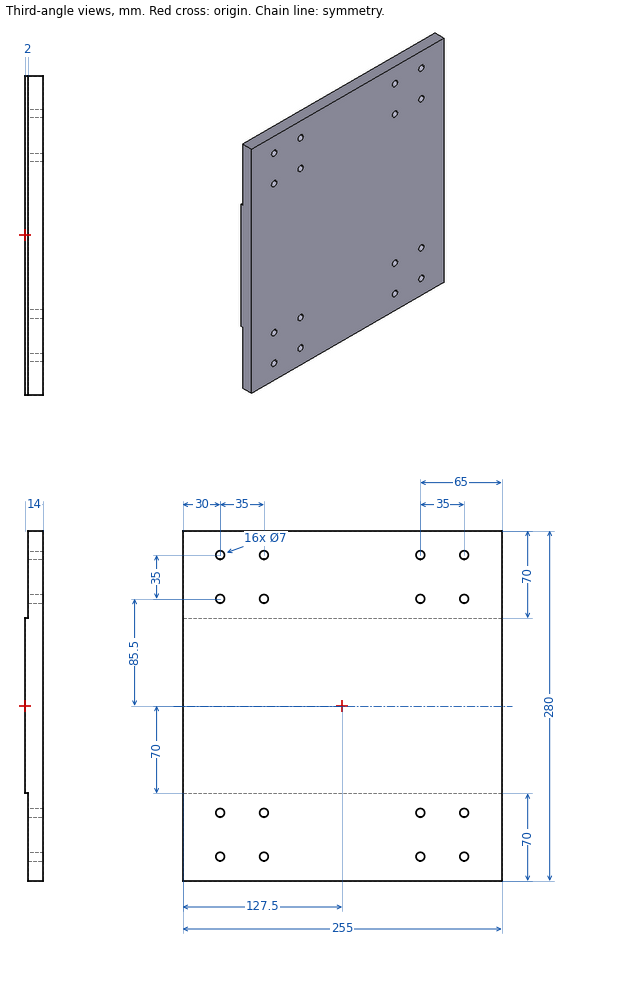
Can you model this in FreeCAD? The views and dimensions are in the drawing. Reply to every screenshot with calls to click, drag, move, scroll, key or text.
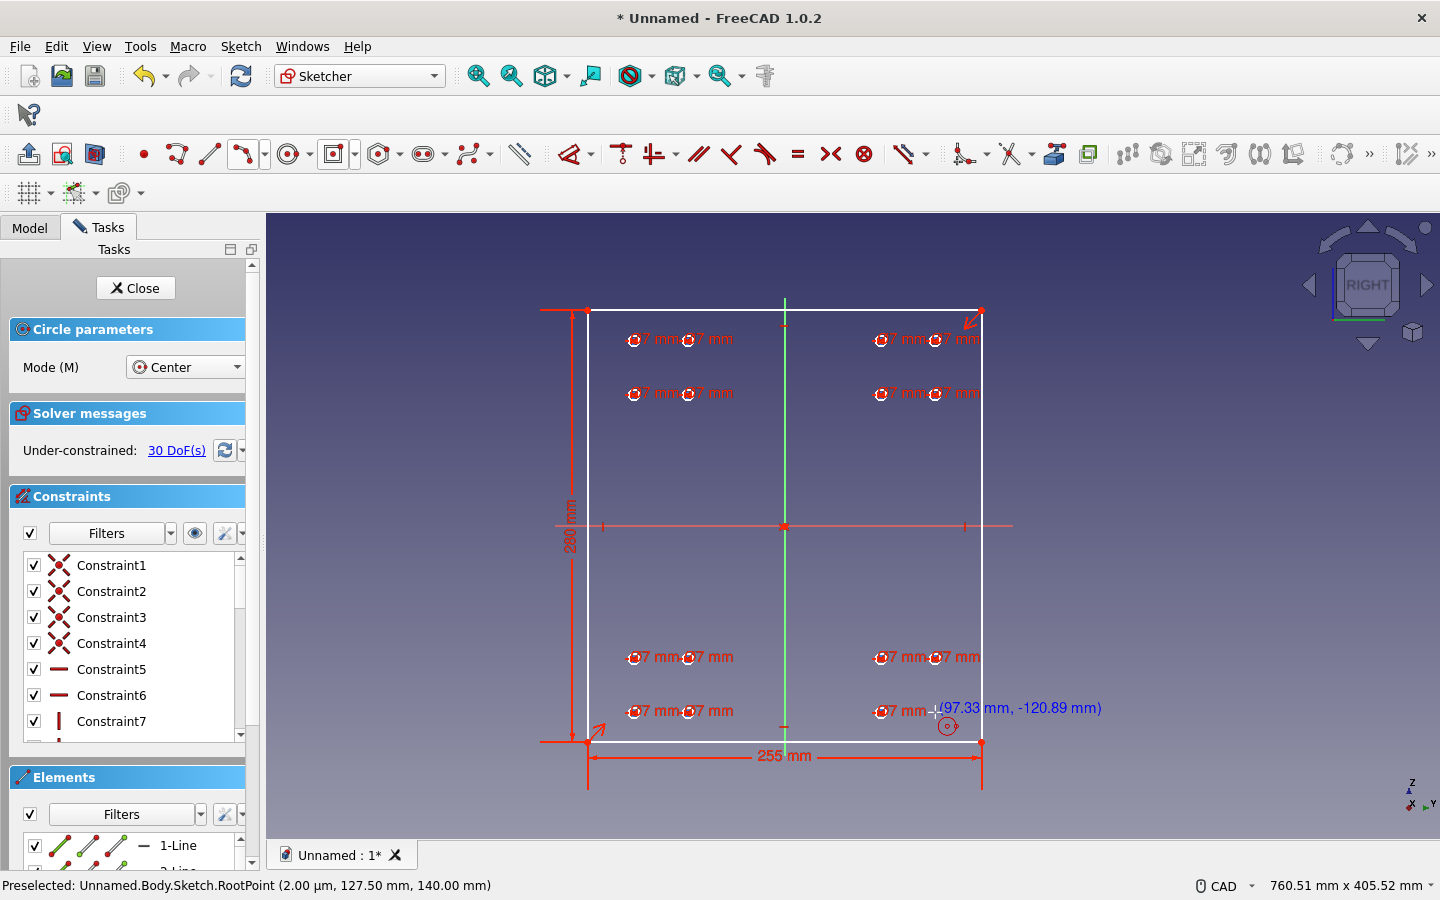
click(935, 712)
move(939, 709)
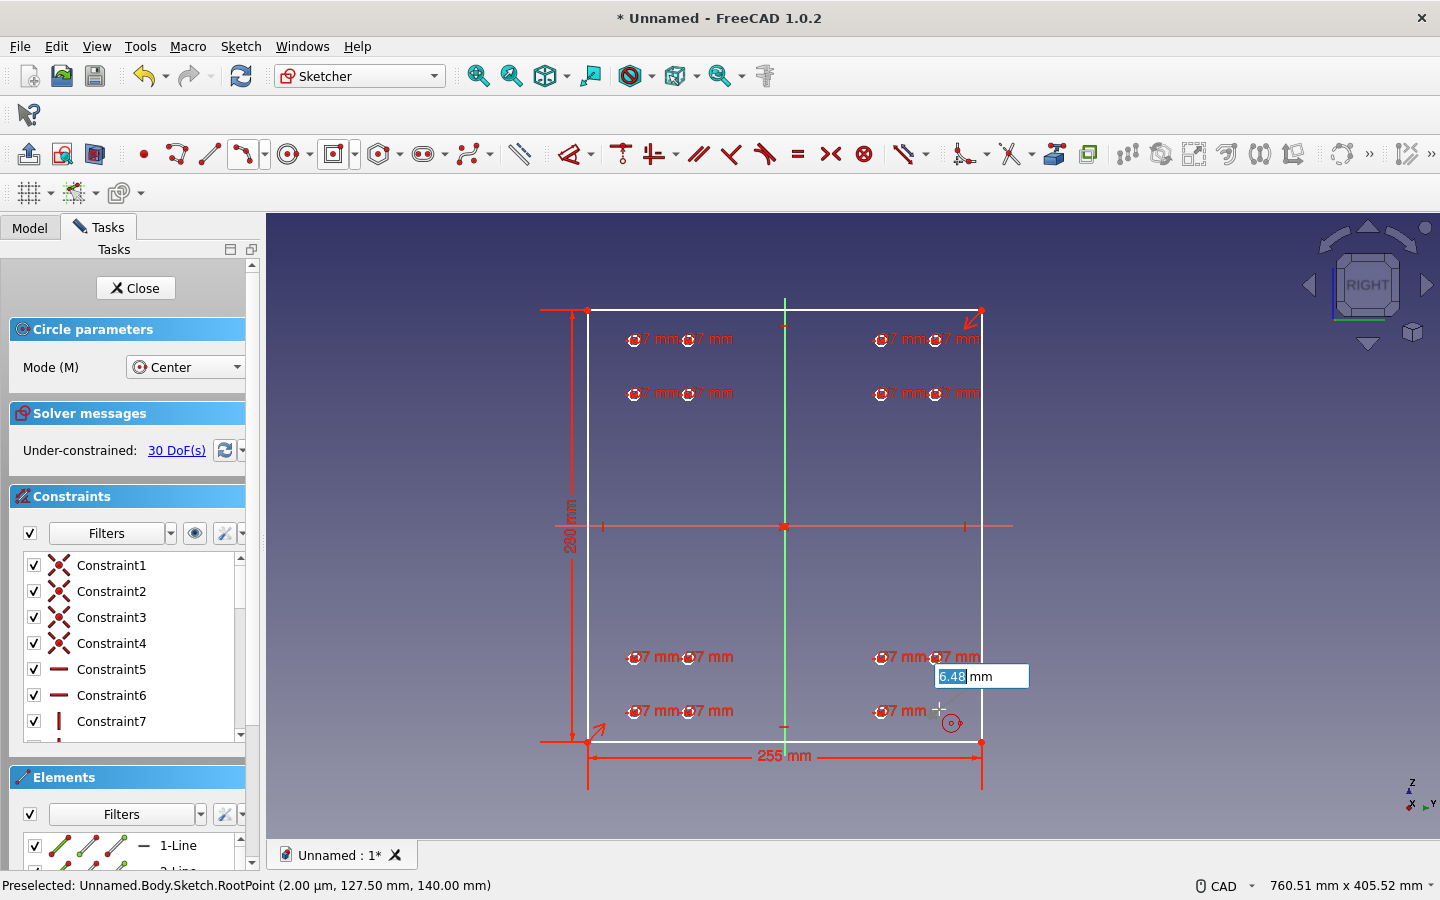
text(7)
key(Return)
key(Escape)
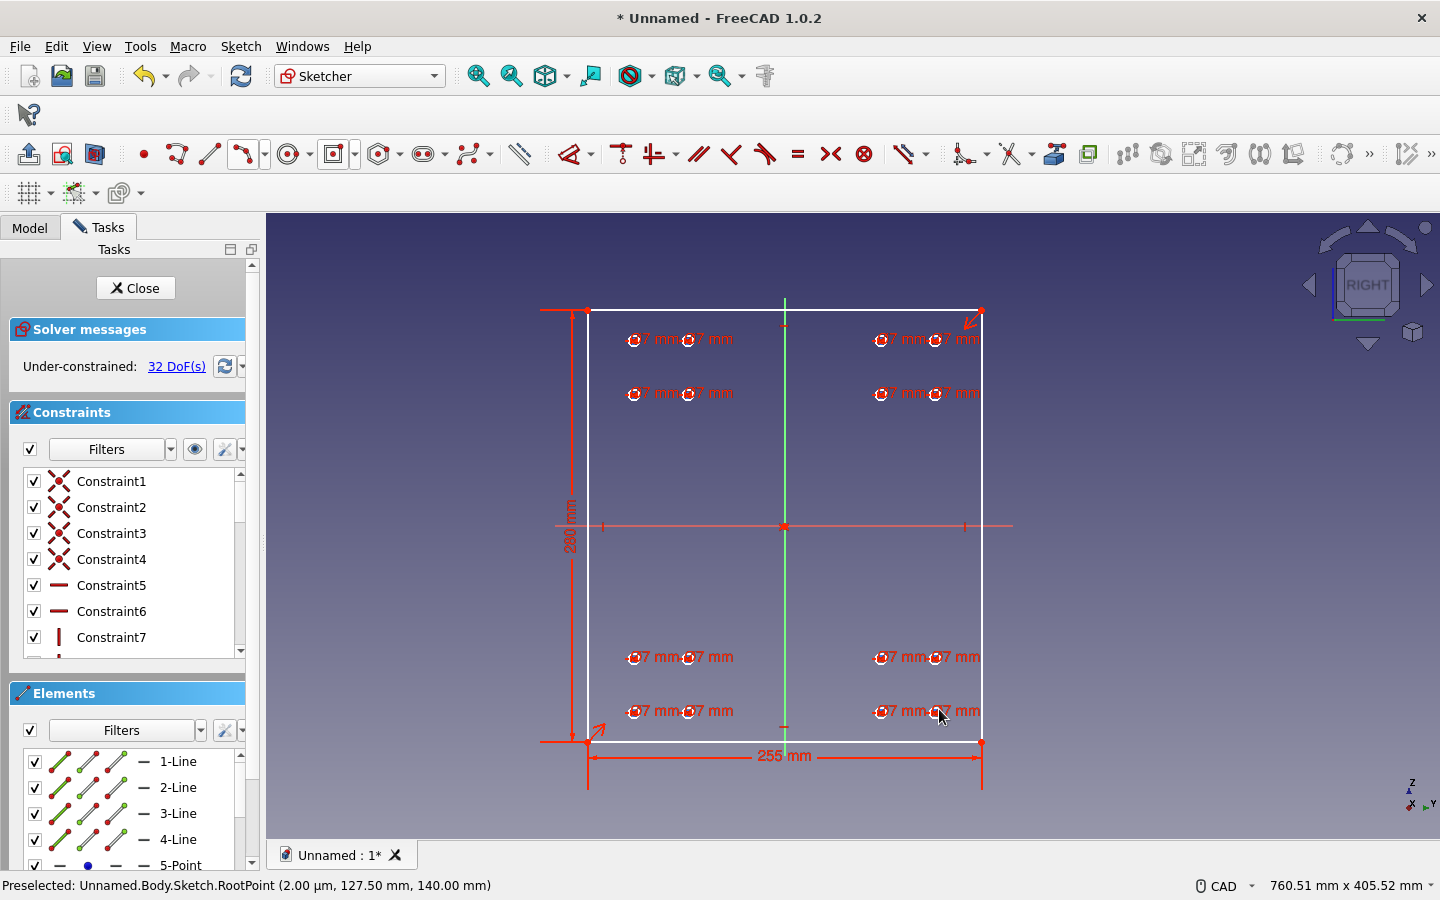
click(634, 341)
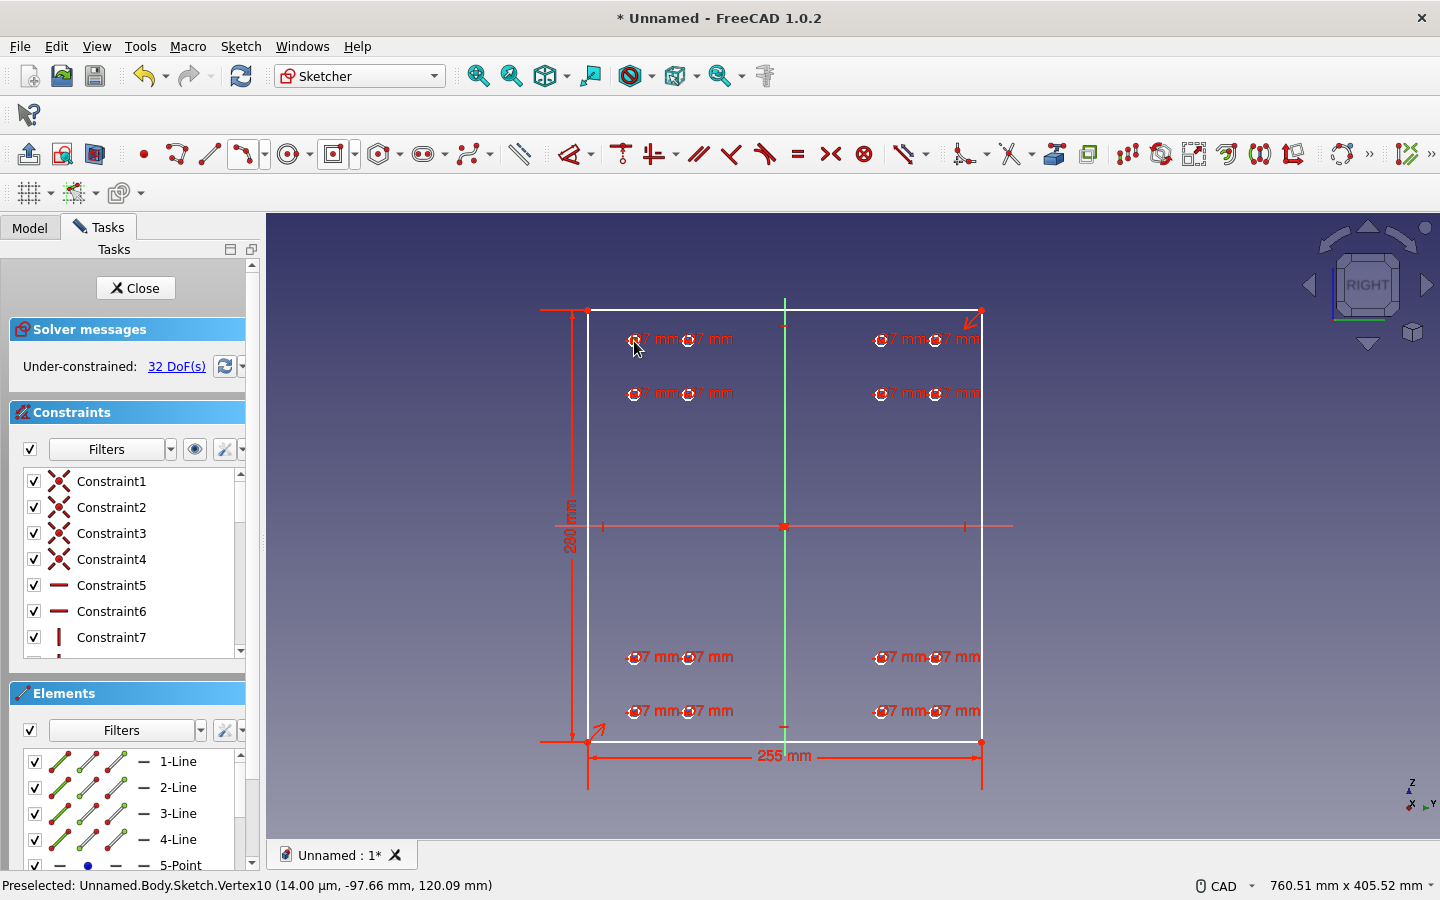
click(634, 395)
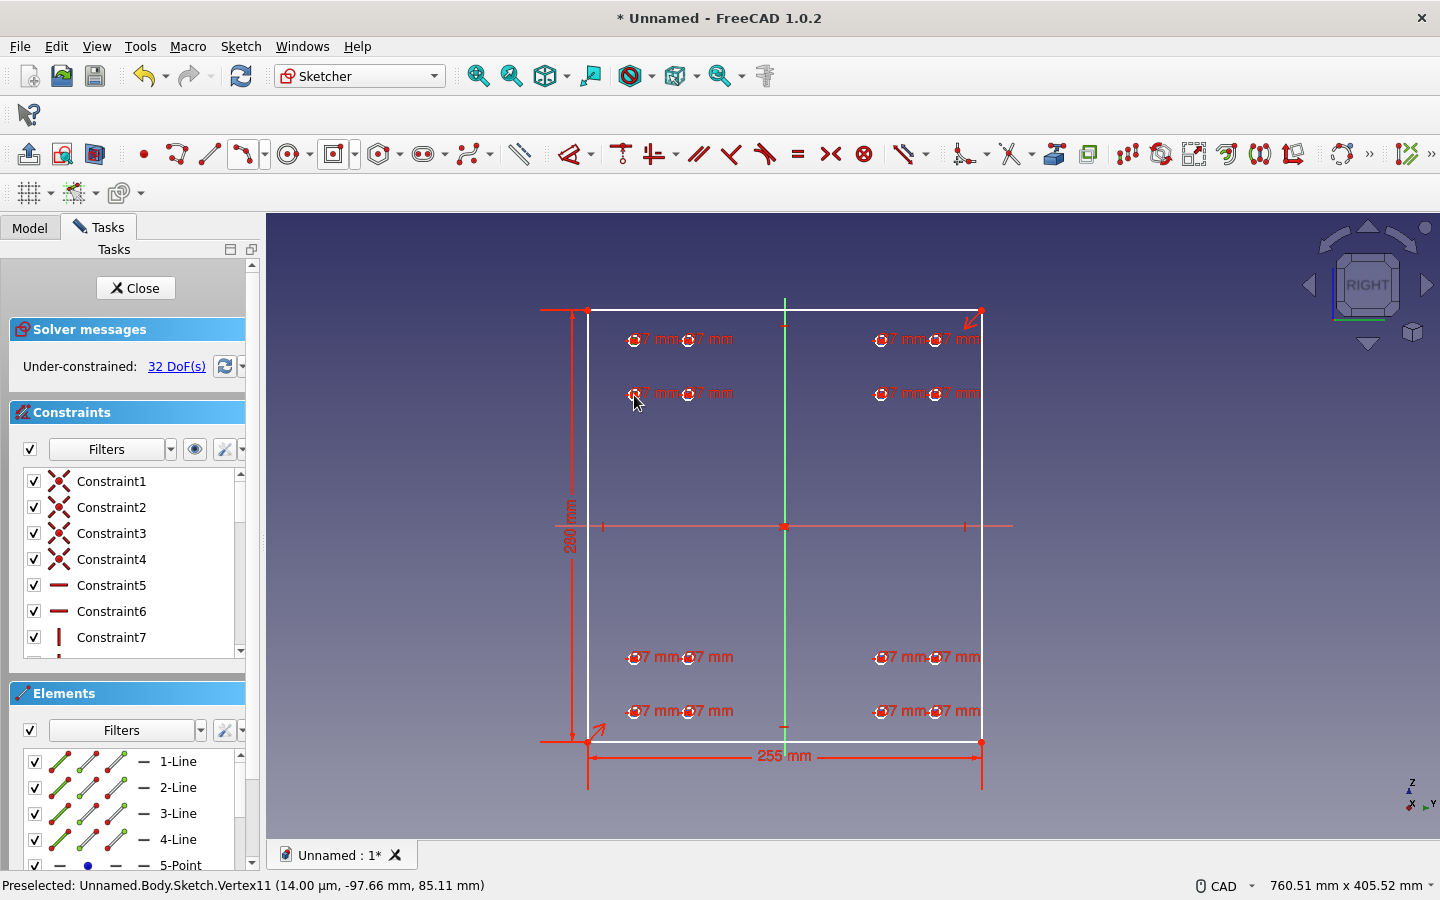
click(676, 154)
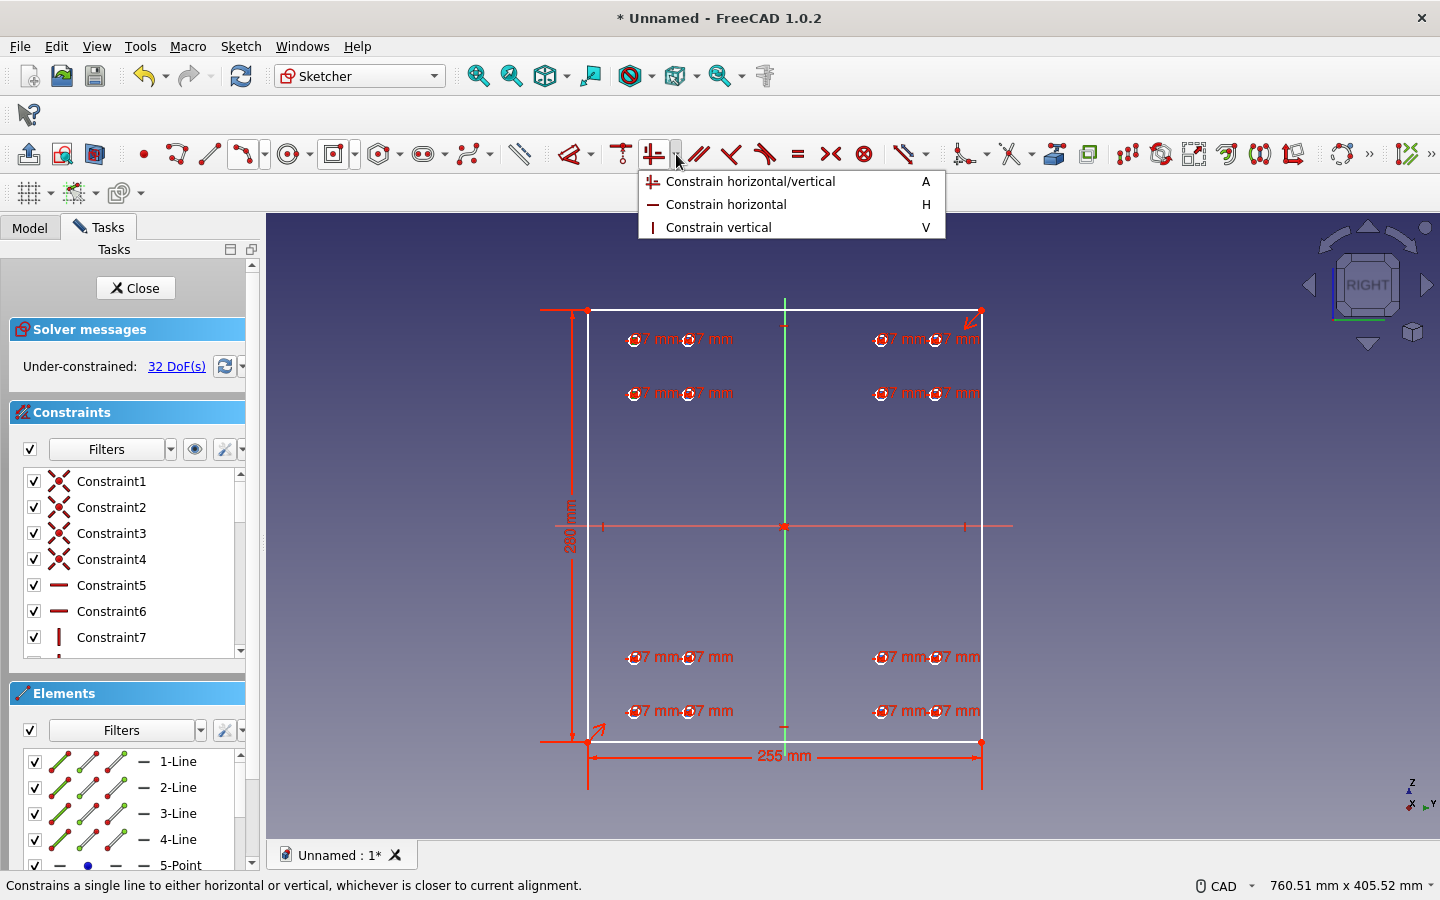
click(792, 228)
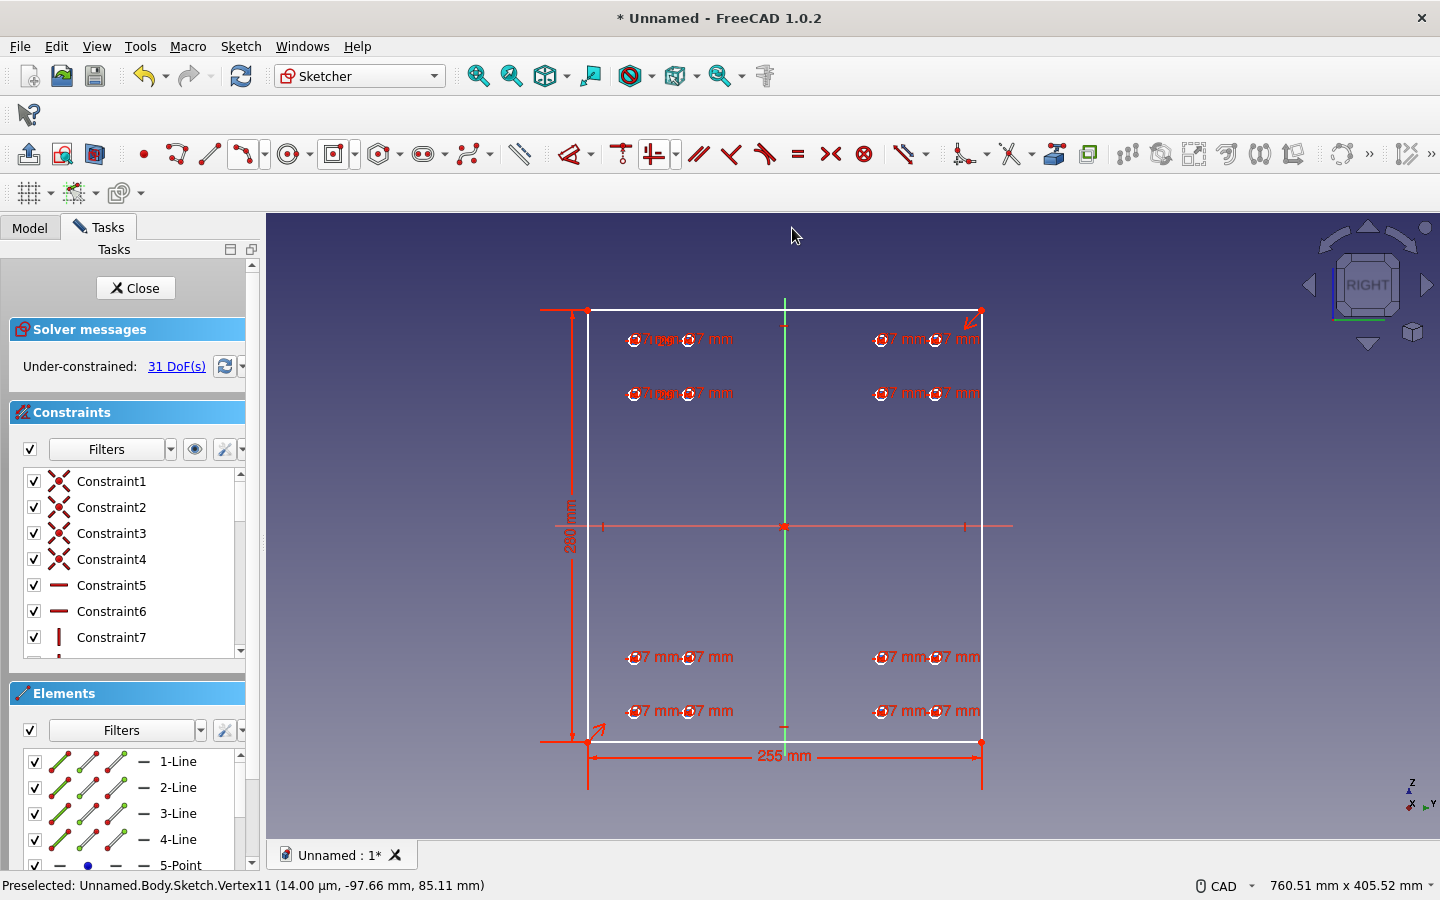
click(634, 341)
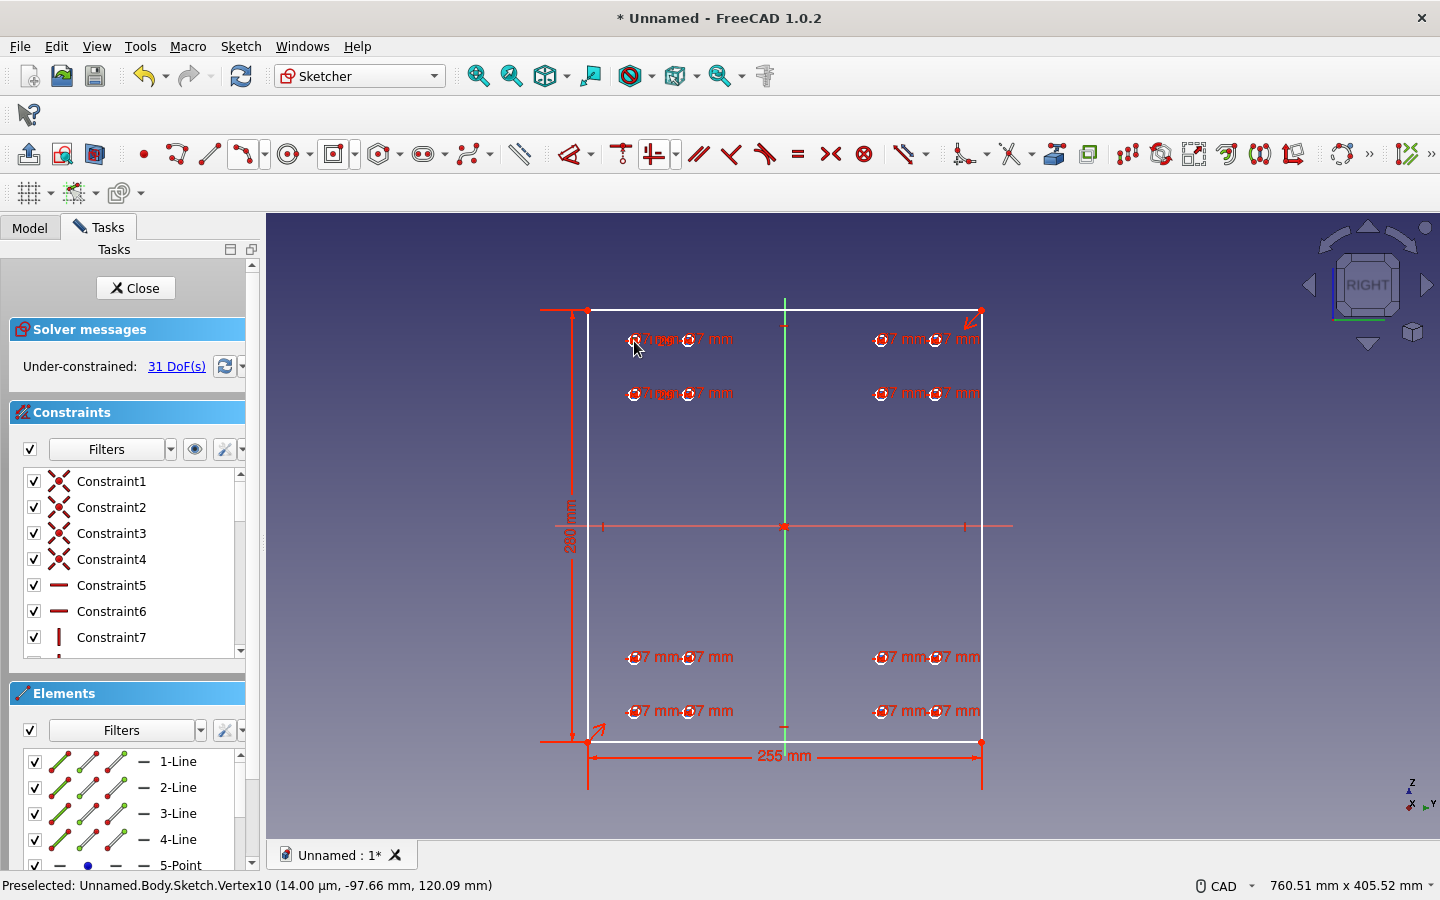
click(688, 341)